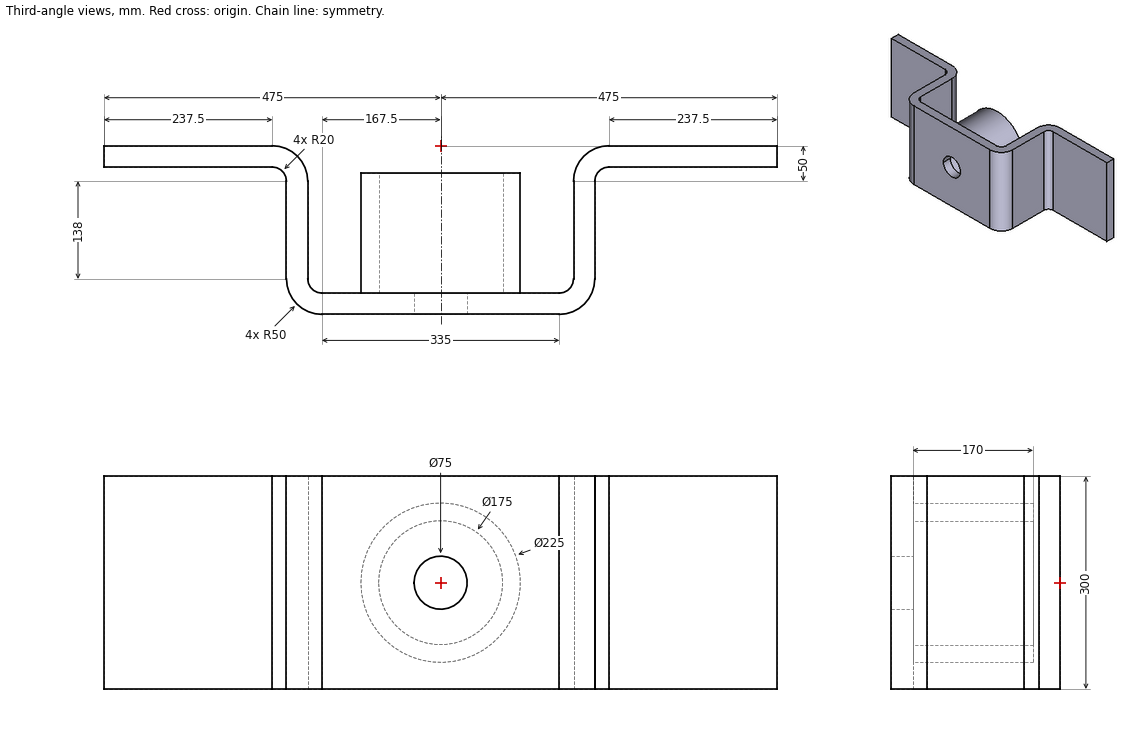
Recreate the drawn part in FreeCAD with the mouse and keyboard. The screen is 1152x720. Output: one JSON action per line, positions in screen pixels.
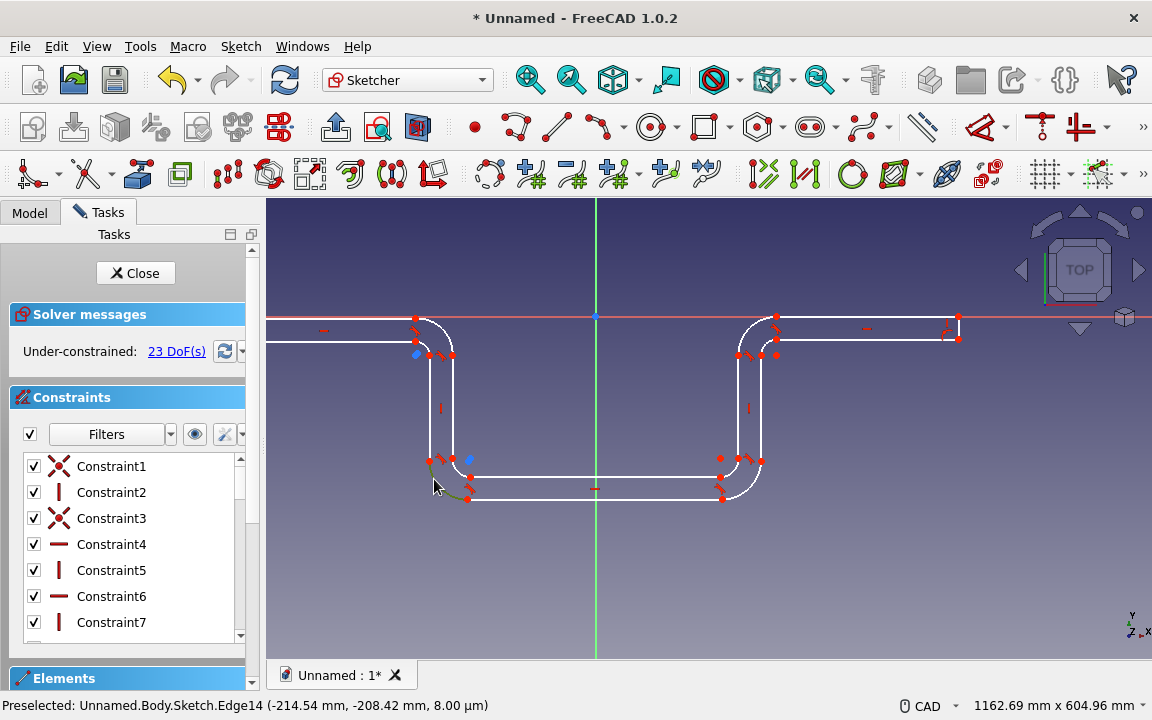
{"action": "left_click", "coordinate": [458, 472]}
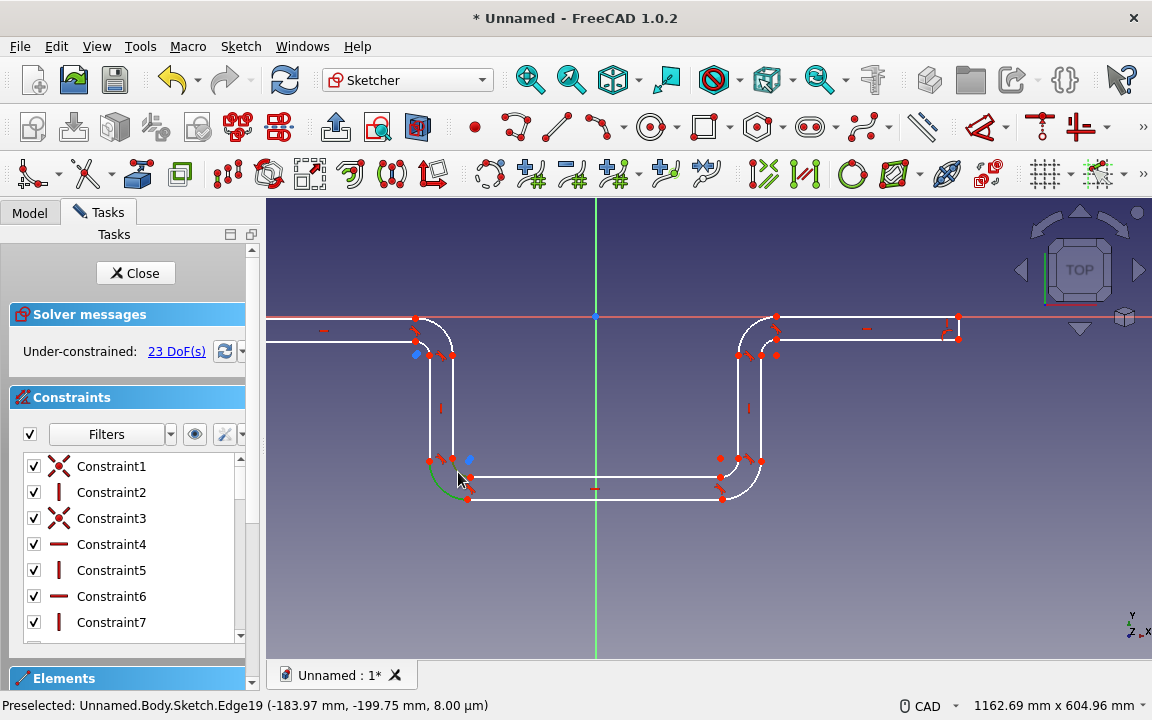
{"action": "key", "text": "c"}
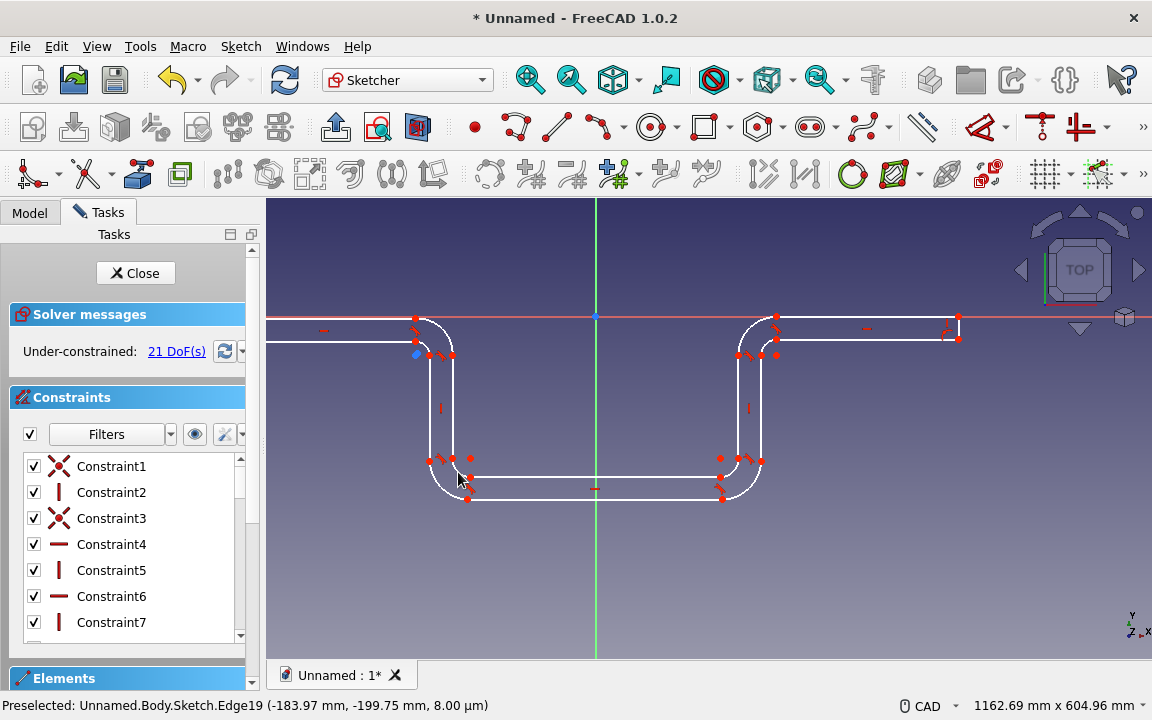
{"action": "scroll", "coordinate": [426, 346], "scroll_direction": "up", "scroll_amount": 2}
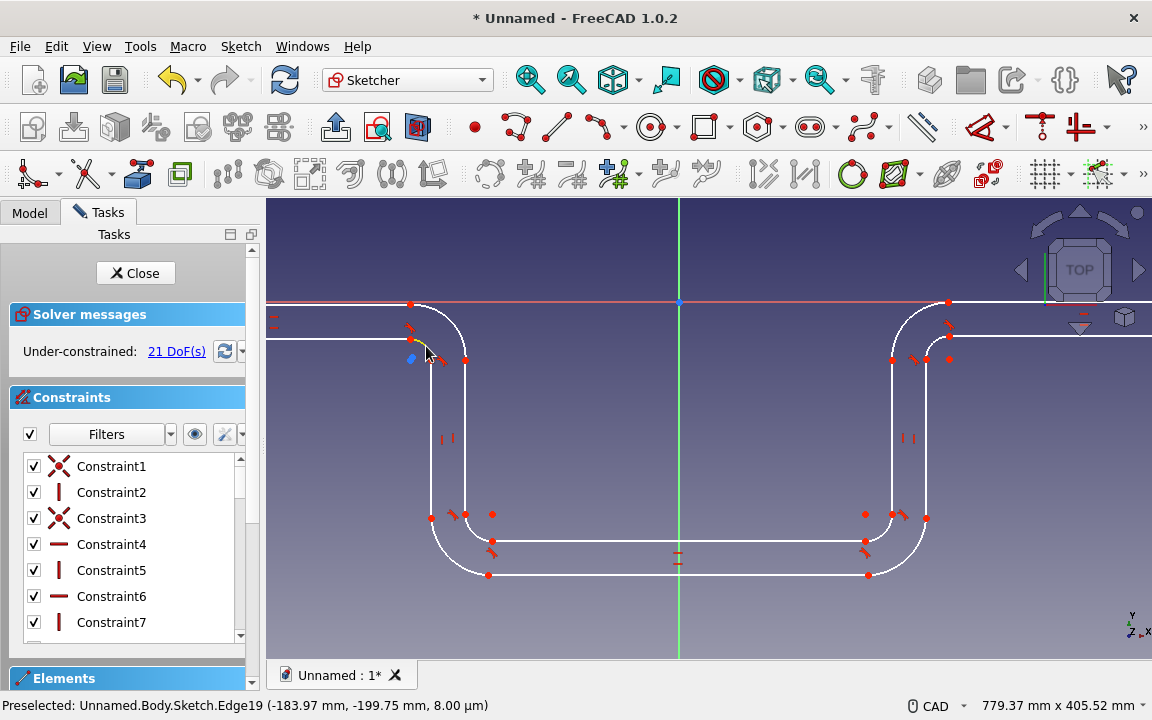
{"action": "left_click", "coordinate": [425, 346]}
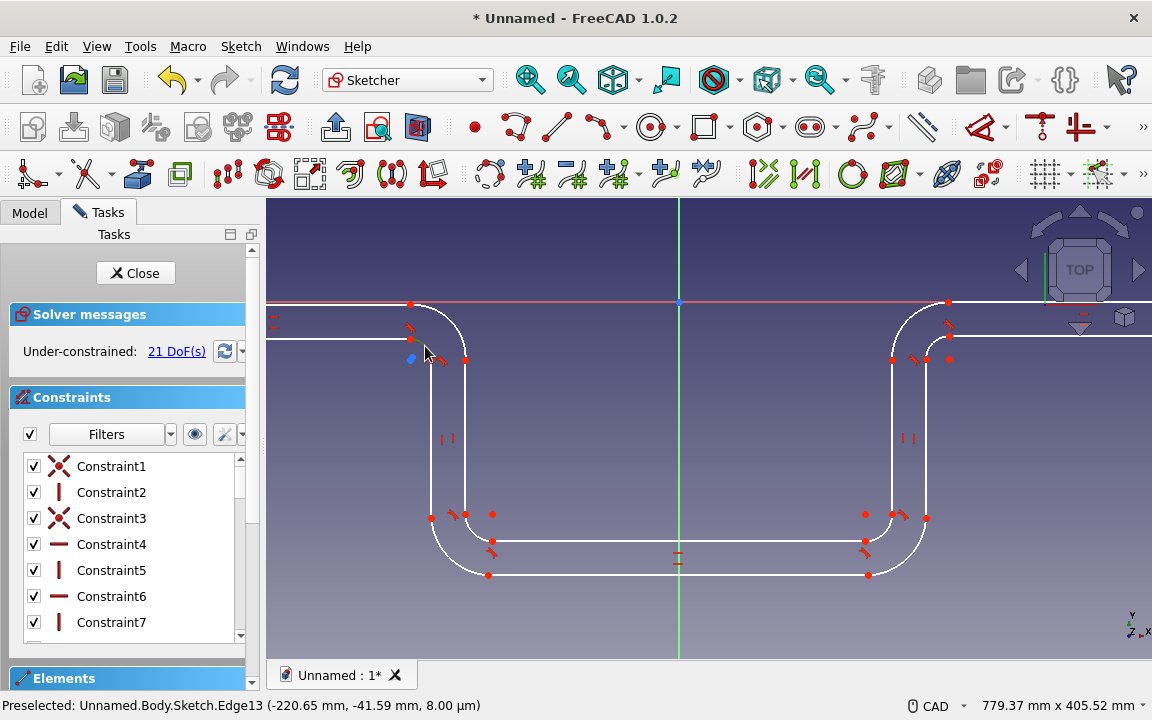
{"action": "left_click", "coordinate": [460, 335]}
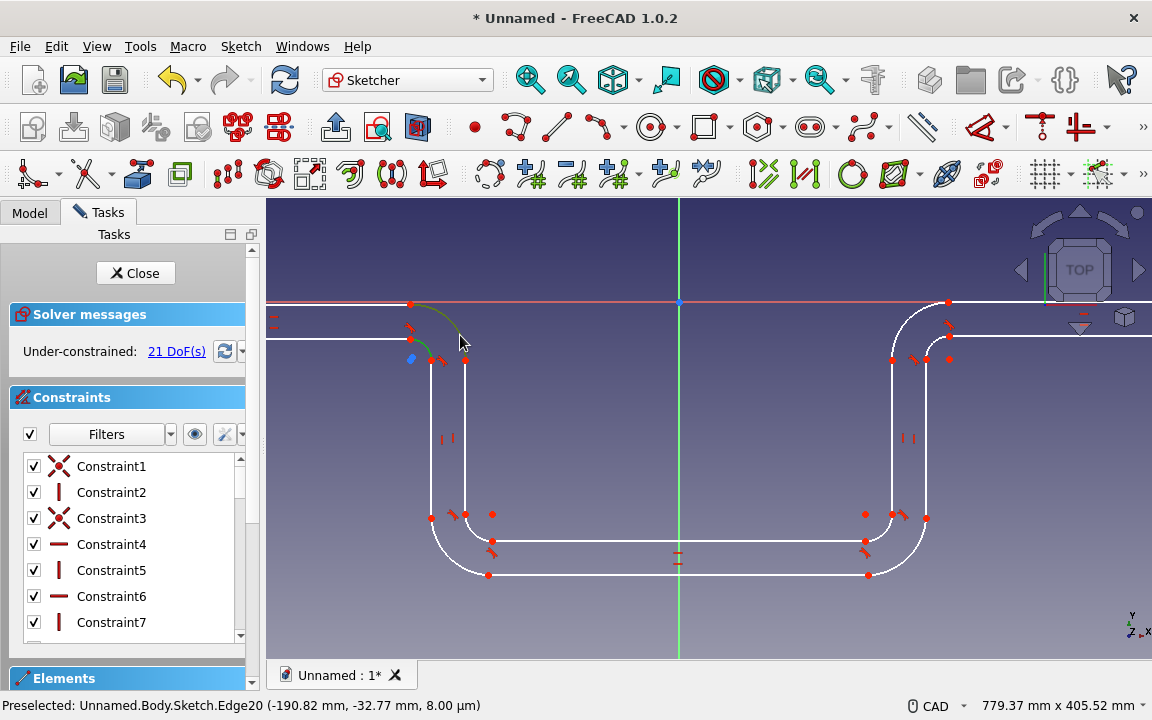
{"action": "key", "text": "c"}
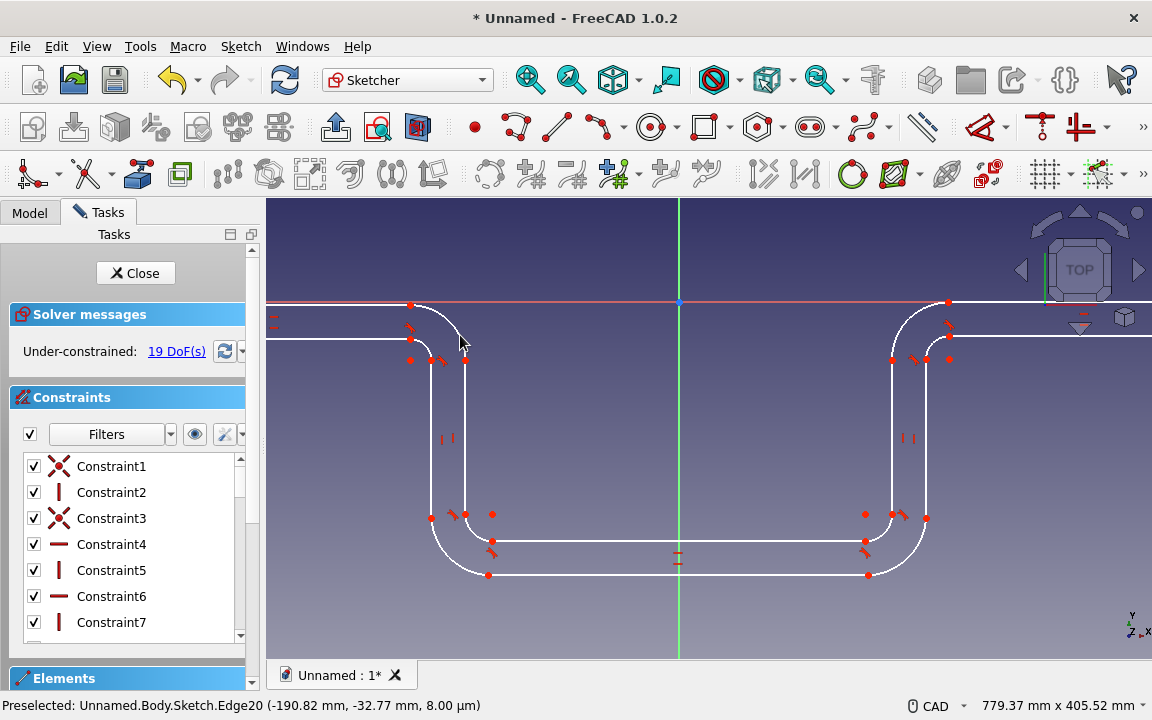
{"action": "left_click", "coordinate": [439, 544]}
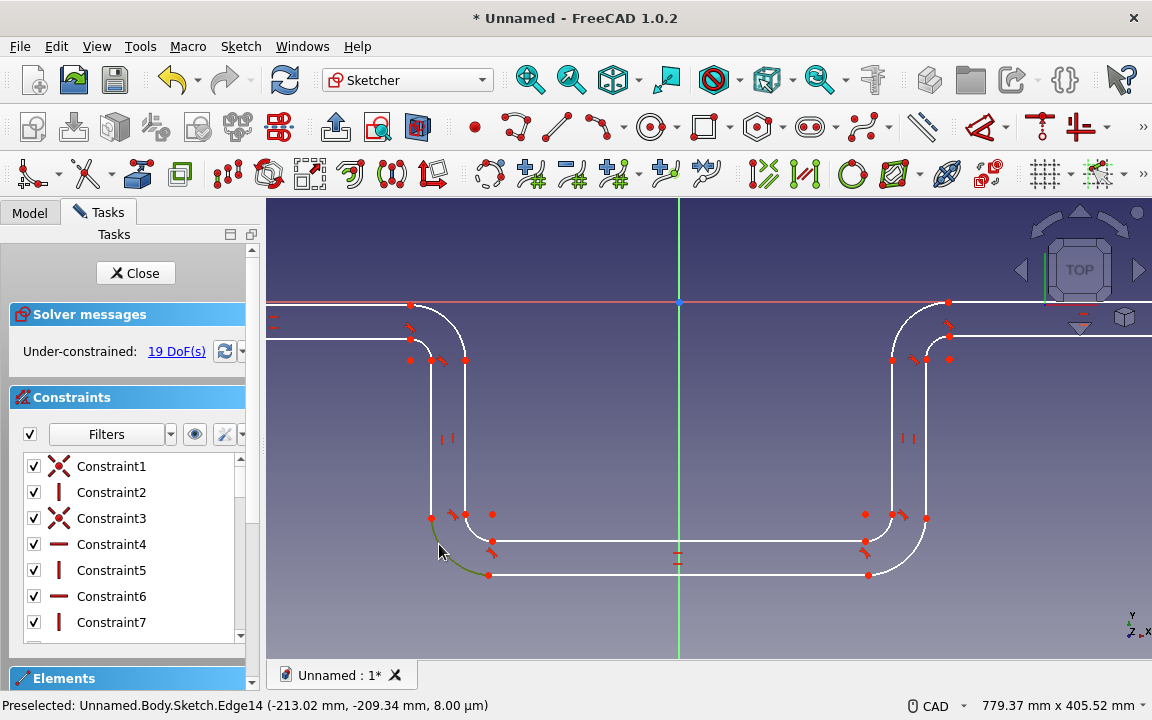
{"action": "left_click", "coordinate": [894, 568]}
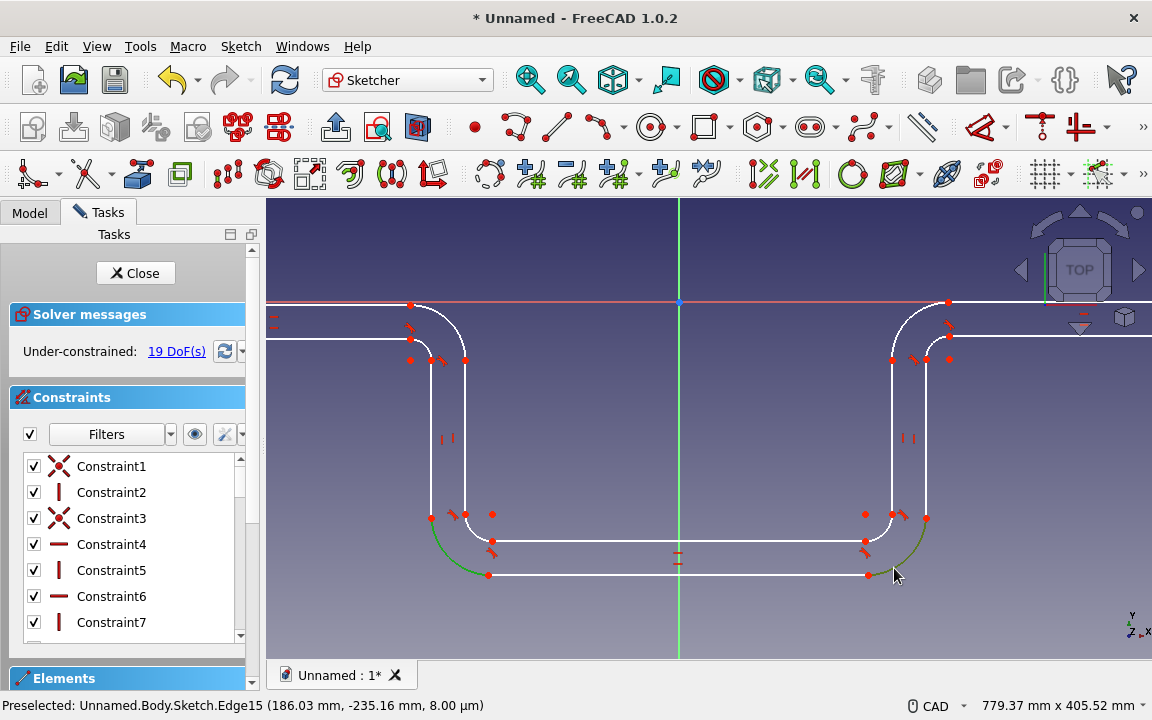
{"action": "left_click", "coordinate": [898, 334]}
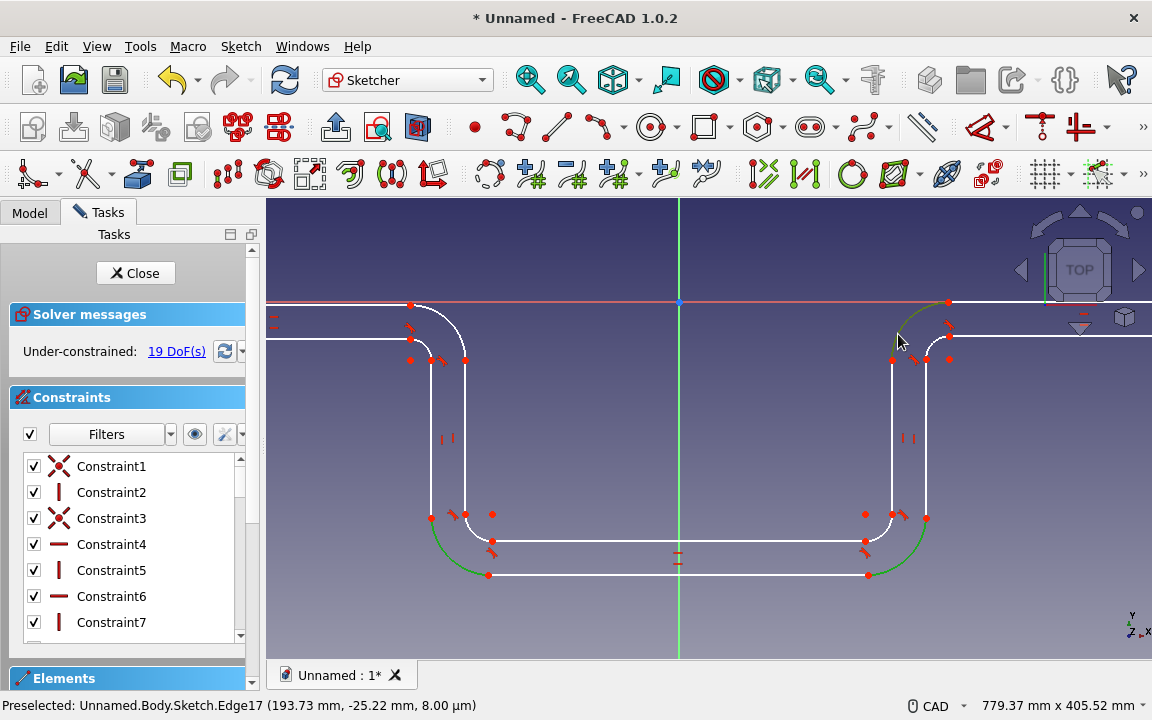
{"action": "left_click", "coordinate": [459, 335]}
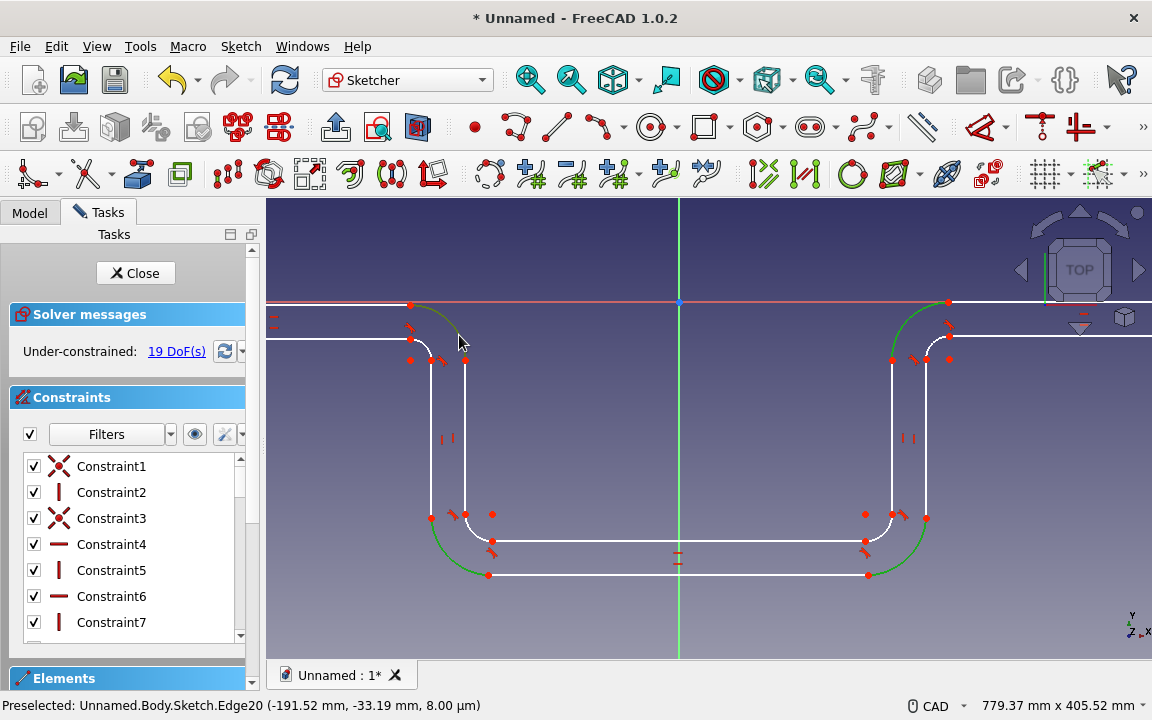
{"action": "key", "text": "e"}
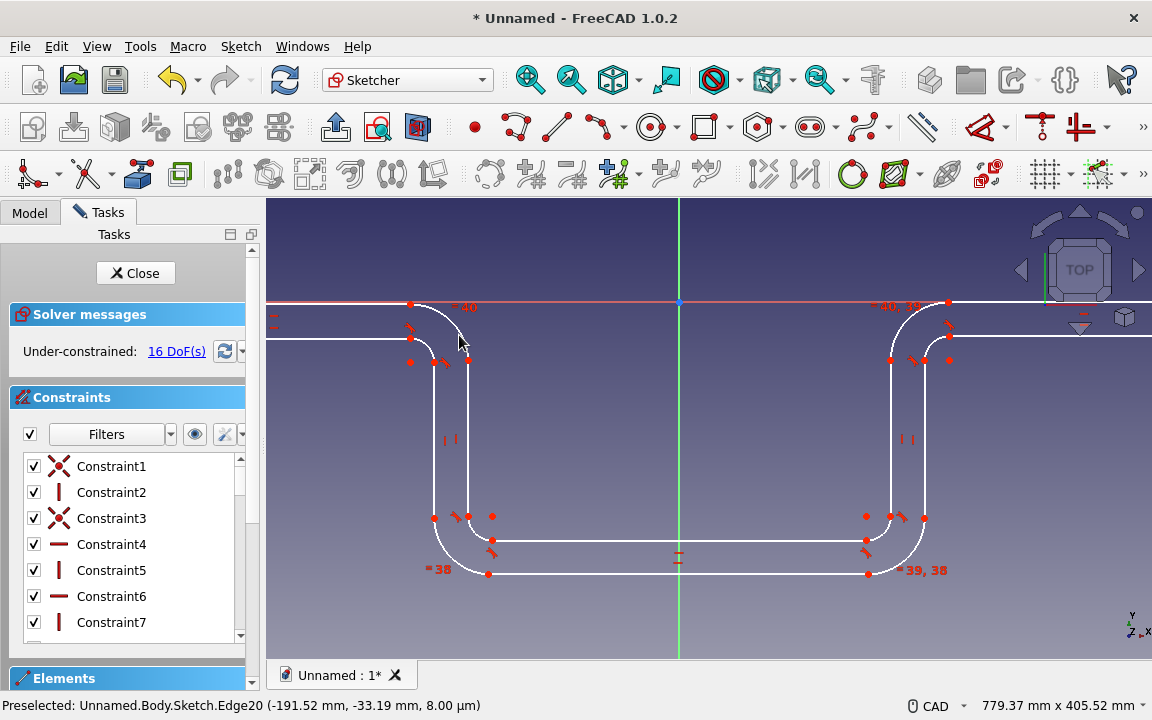
{"action": "left_click", "coordinate": [410, 363]}